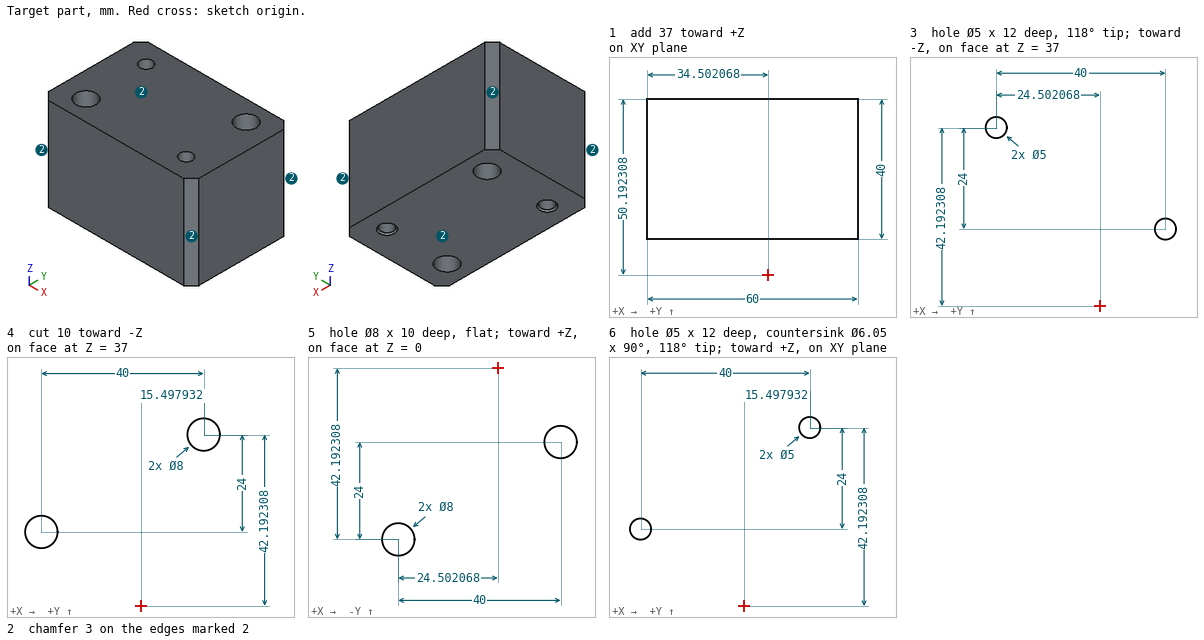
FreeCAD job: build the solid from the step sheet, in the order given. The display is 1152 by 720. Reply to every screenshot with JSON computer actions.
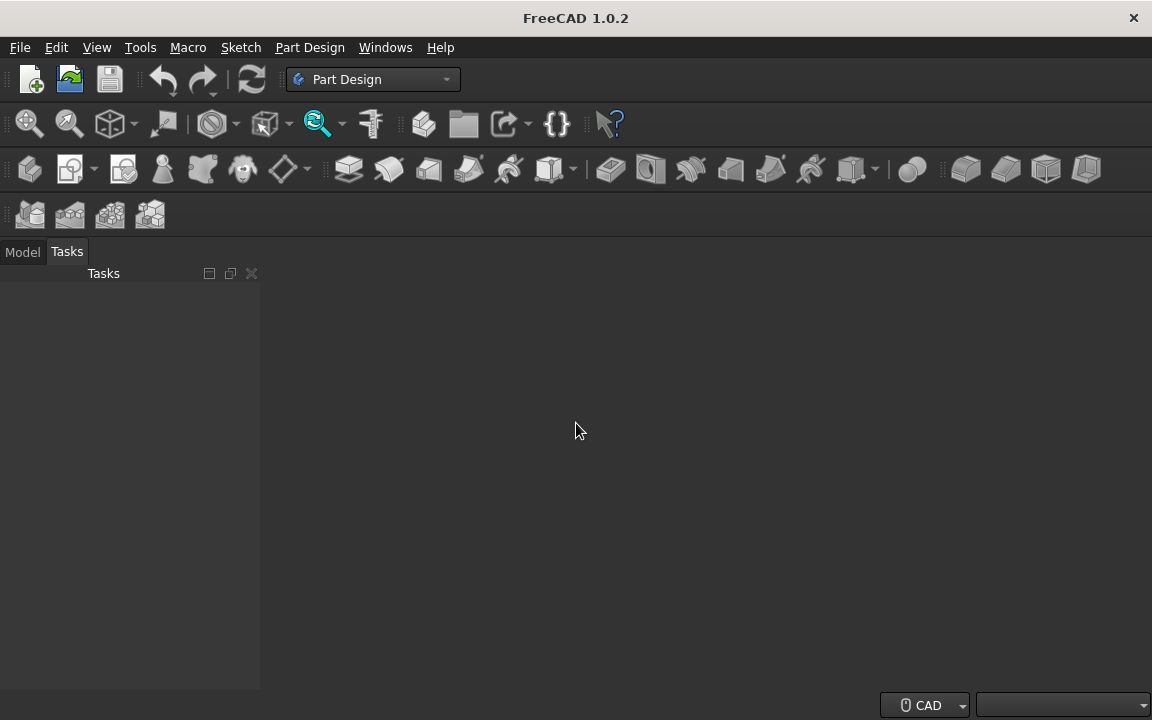
{"action": "left_click", "coordinate": [30, 80]}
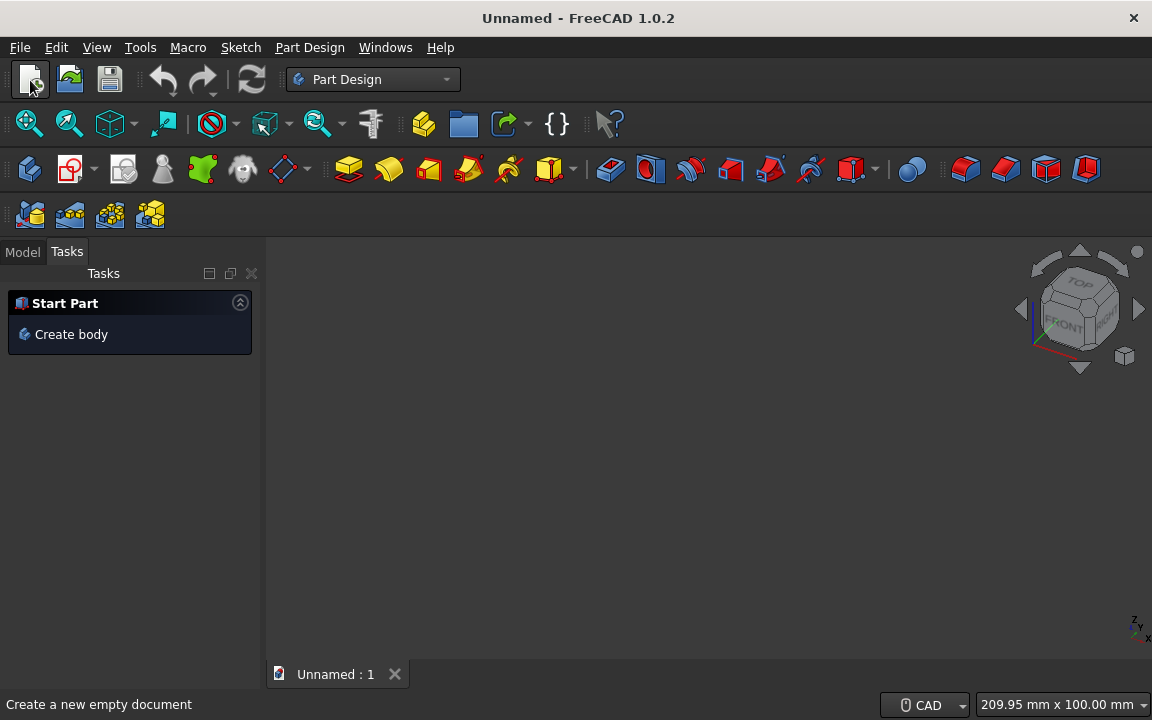
{"action": "left_click", "coordinate": [70, 170]}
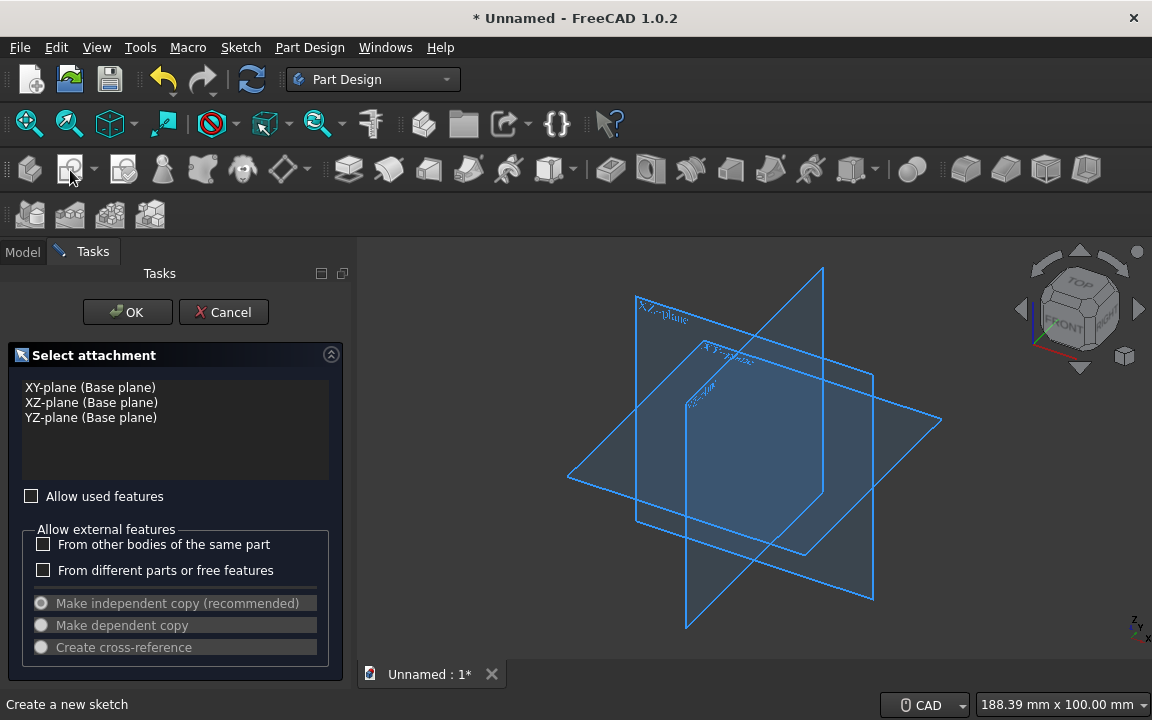
{"action": "left_click", "coordinate": [82, 388]}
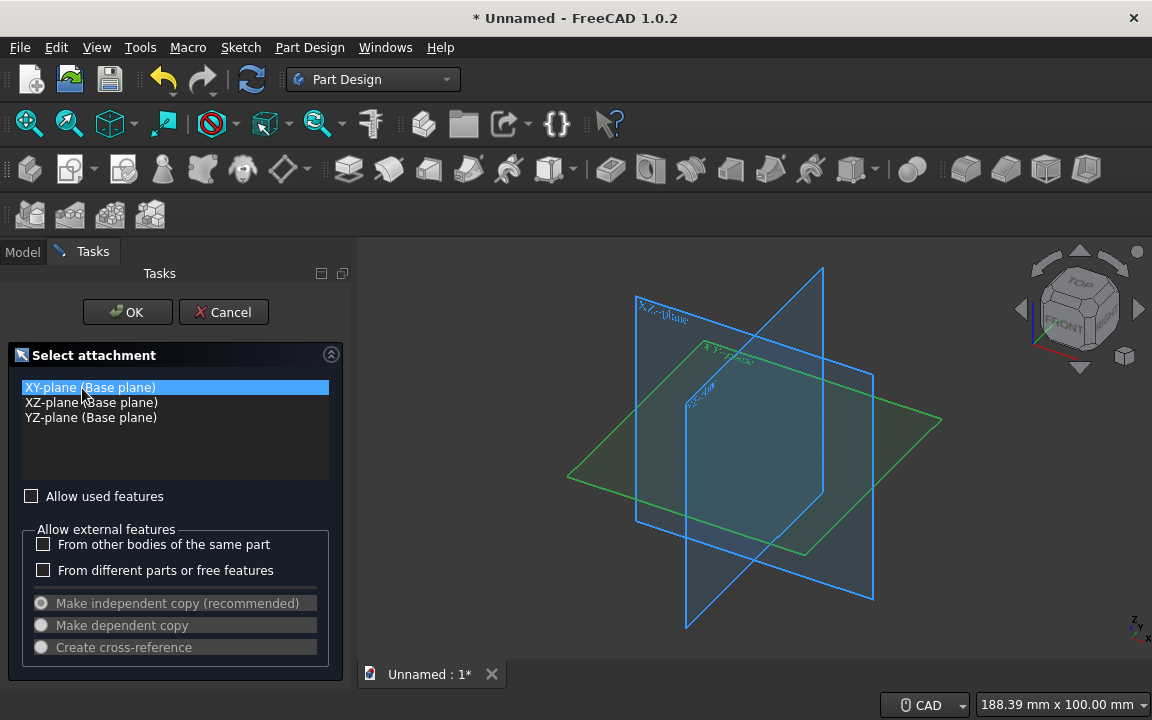
{"action": "left_click", "coordinate": [128, 312]}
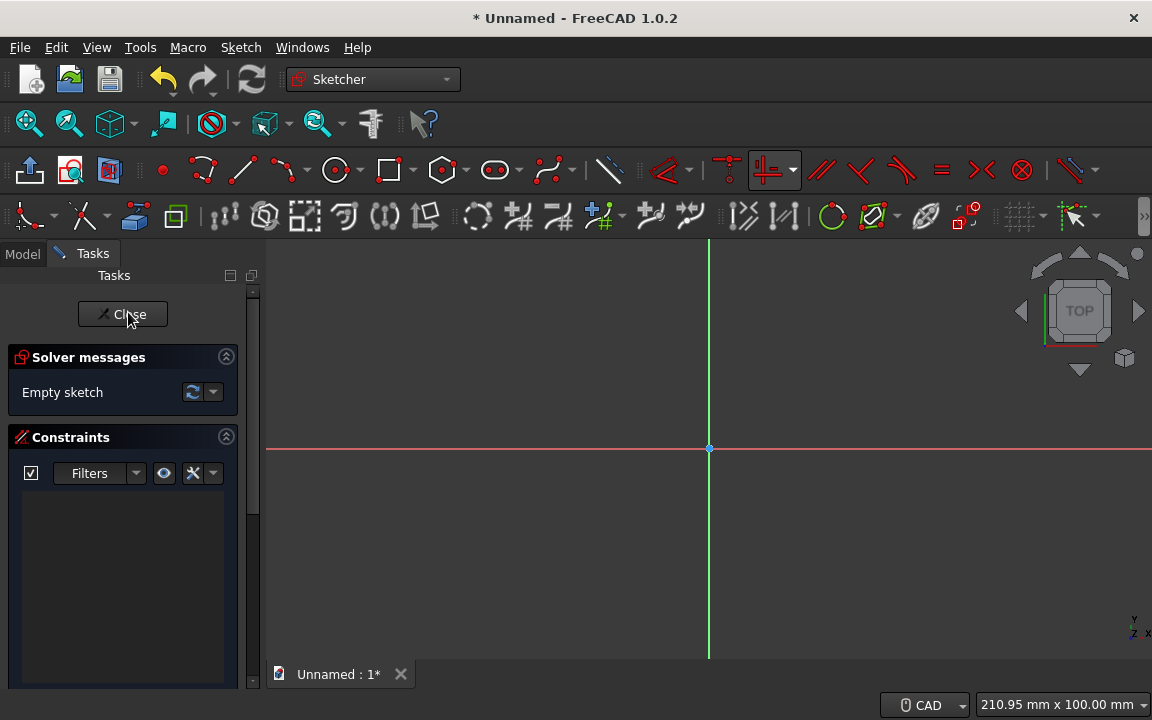
{"action": "scroll", "coordinate": [417, 631], "scroll_direction": "down", "scroll_amount": 1}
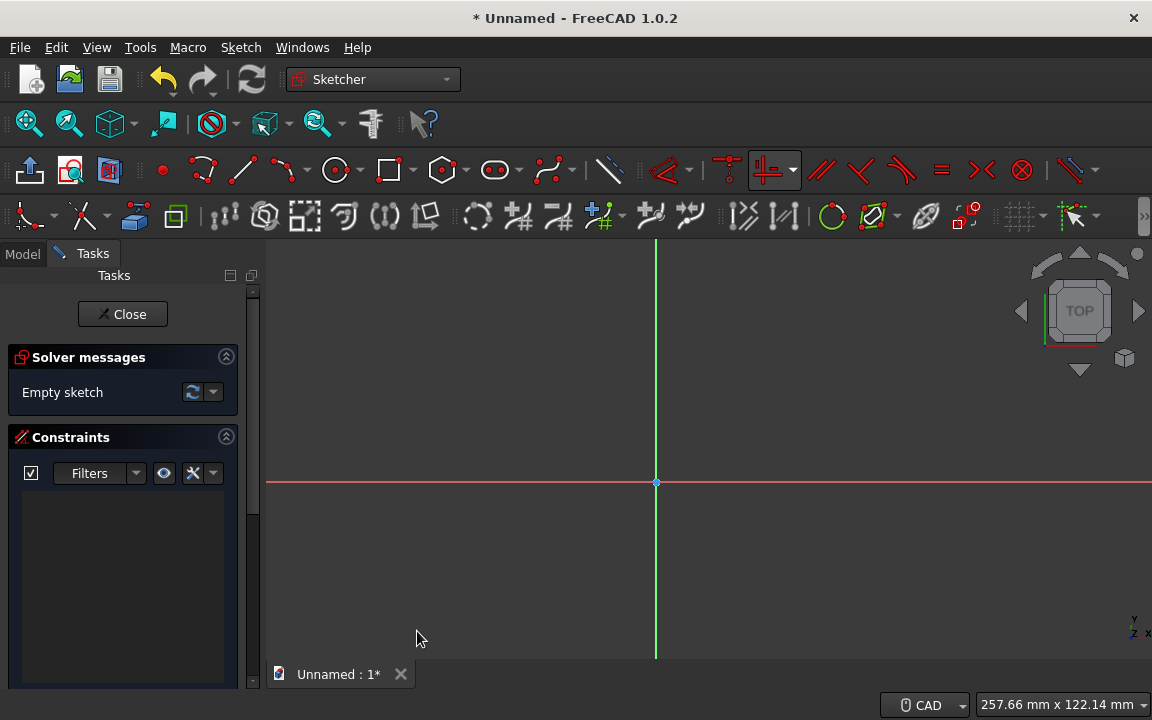
{"action": "scroll", "coordinate": [641, 288], "scroll_direction": "up", "scroll_amount": 2}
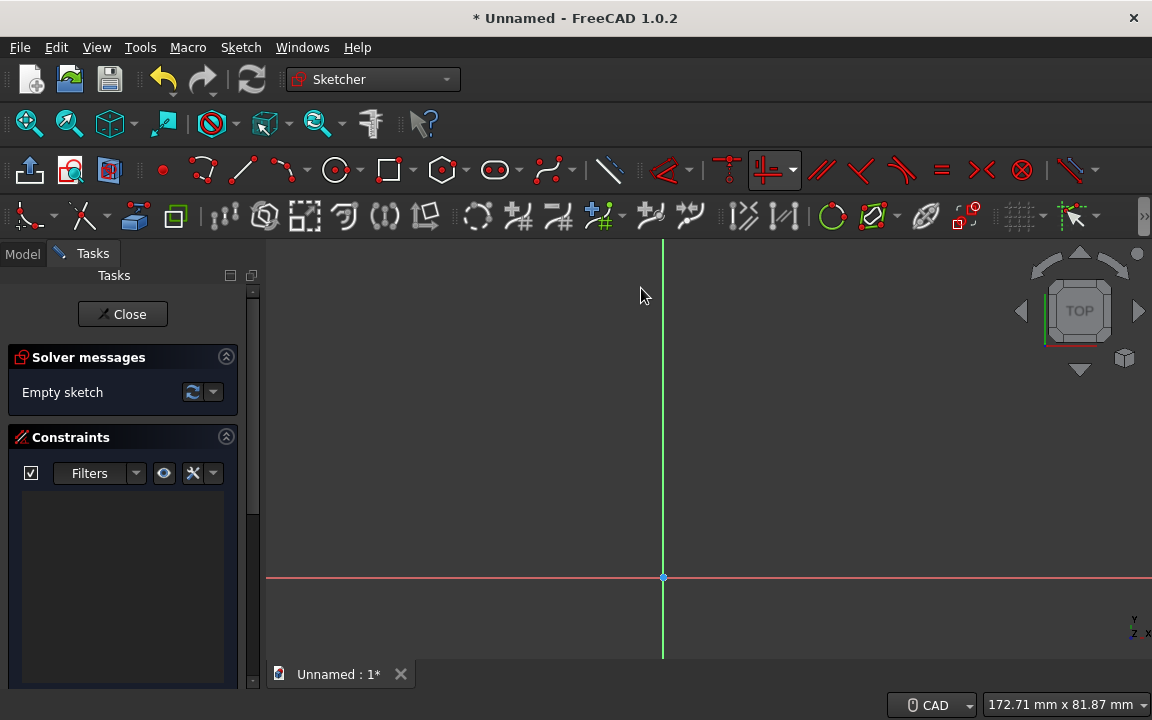
{"action": "left_click", "coordinate": [390, 170]}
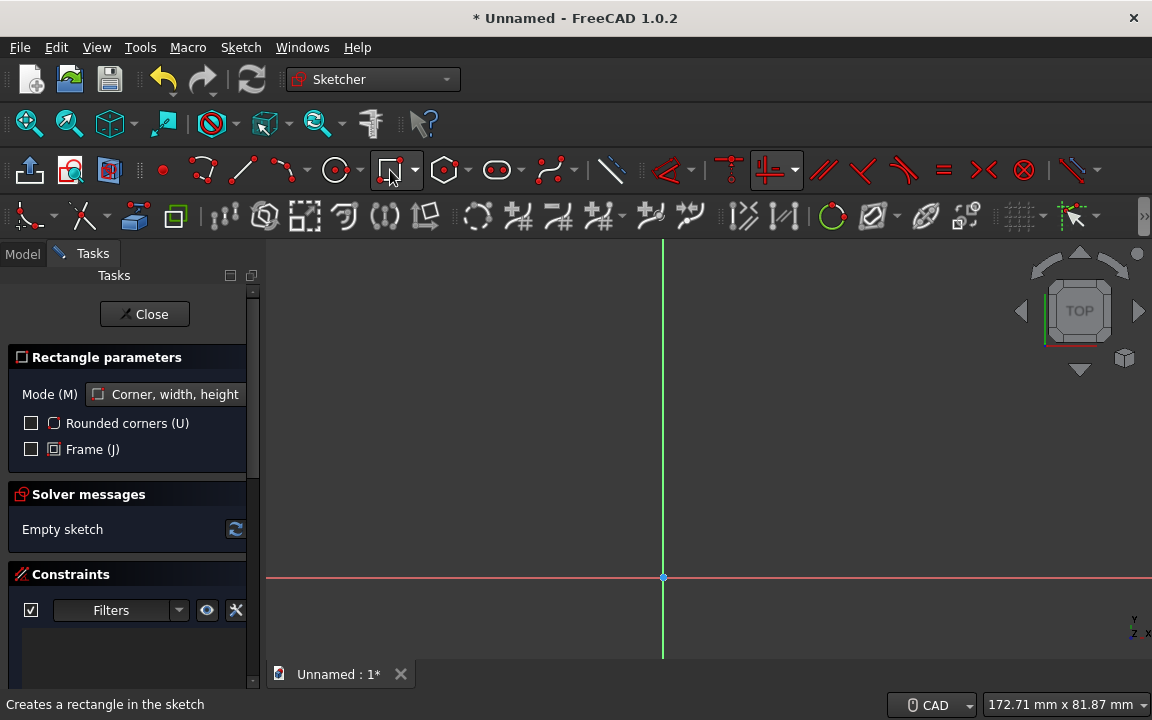
{"action": "left_click", "coordinate": [486, 320]}
{"action": "mouse_move", "coordinate": [794, 525]}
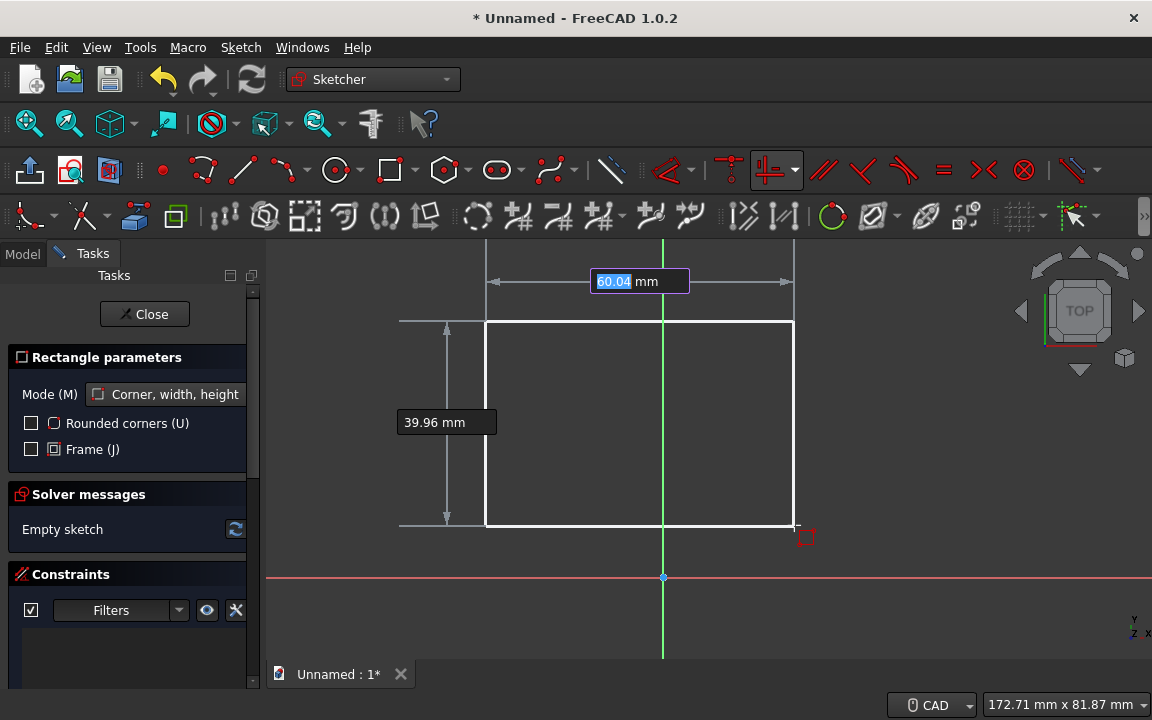
{"action": "type", "text": "60"}
{"action": "key", "text": "Tab"}
{"action": "type", "text": "40"}
{"action": "key", "text": "Return"}
{"action": "key", "text": "Escape"}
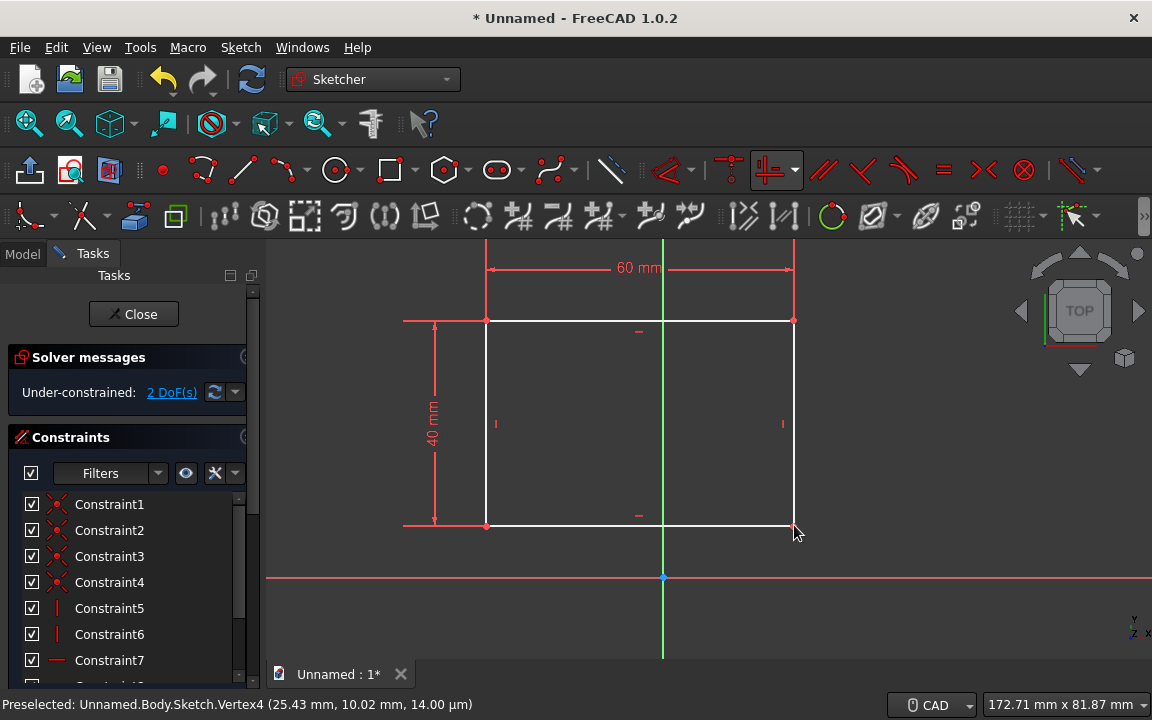
{"action": "left_click", "coordinate": [666, 170]}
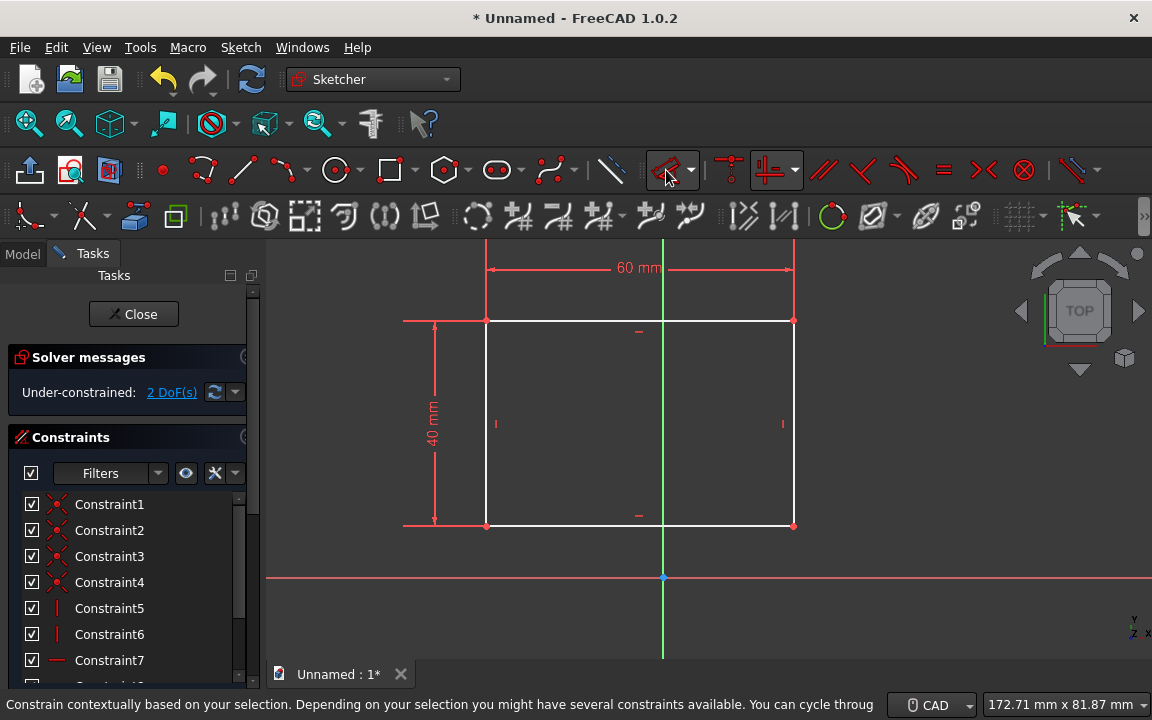
{"action": "left_click", "coordinate": [486, 321]}
{"action": "left_click", "coordinate": [575, 612]}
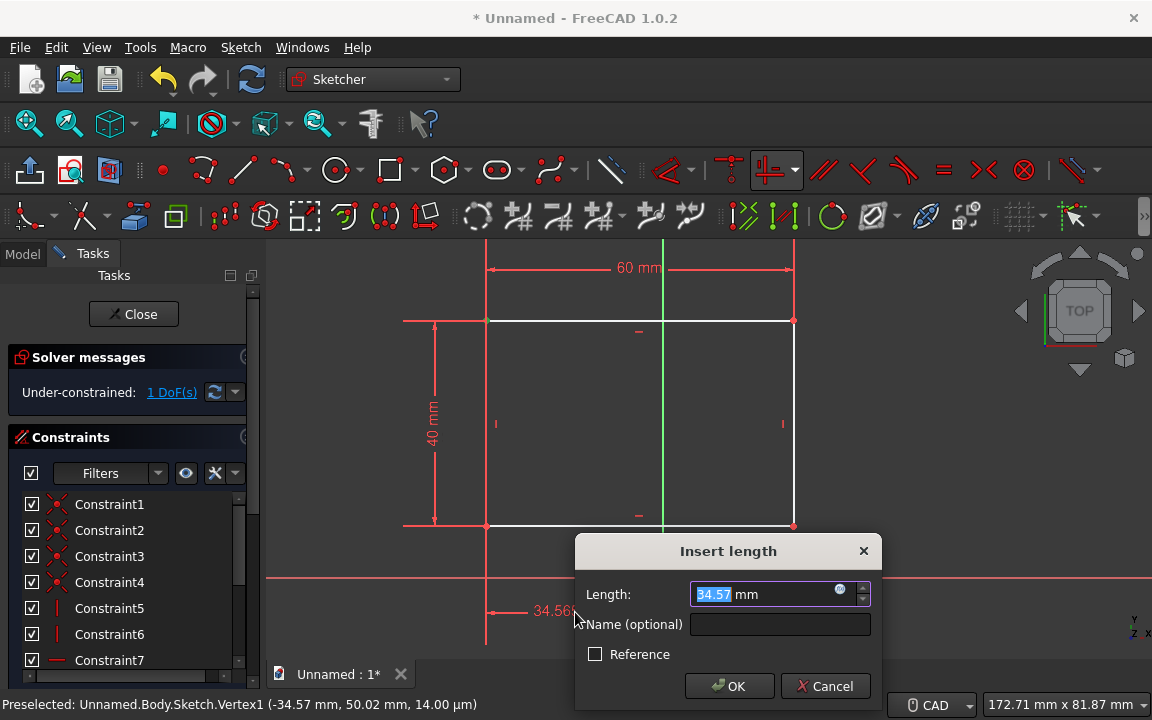
{"action": "type", "text": "34.502068"}
{"action": "key", "text": "Return"}